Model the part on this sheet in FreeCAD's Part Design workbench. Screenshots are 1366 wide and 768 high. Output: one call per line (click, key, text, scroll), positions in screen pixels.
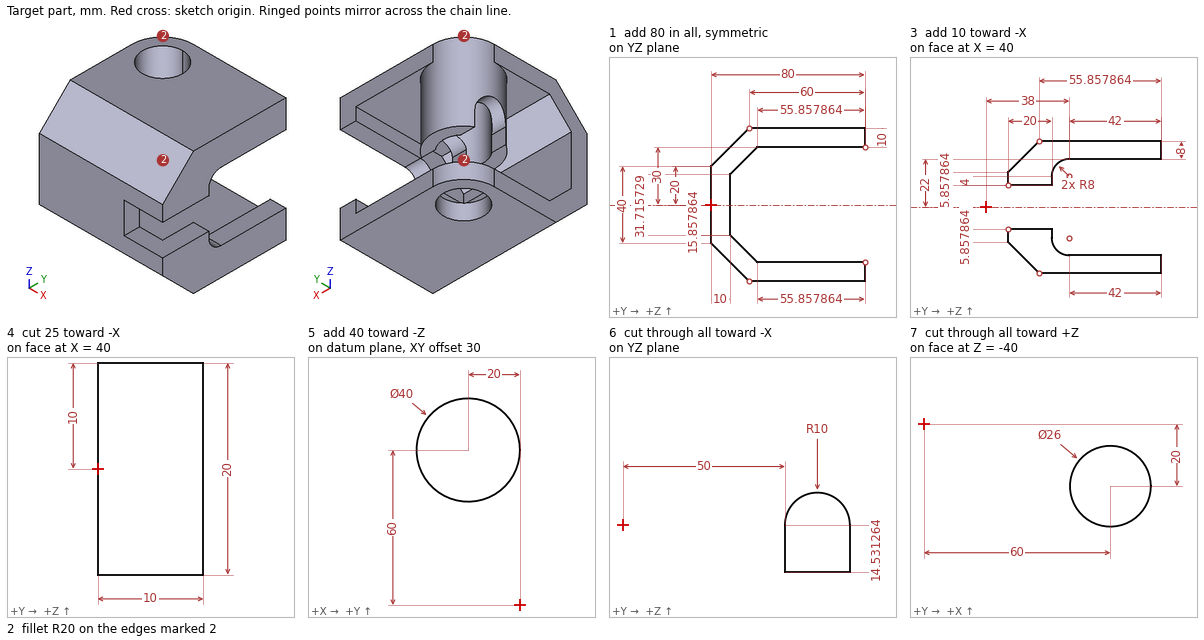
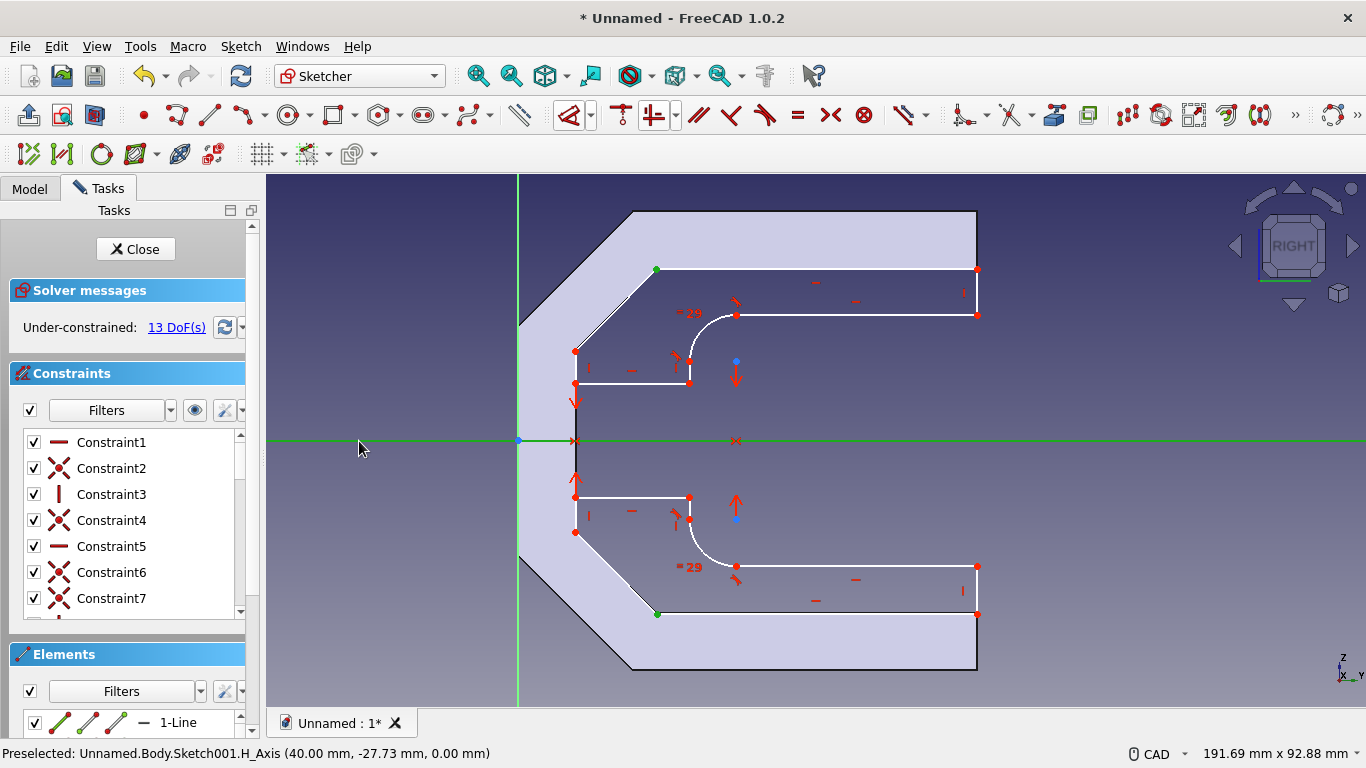
click(831, 116)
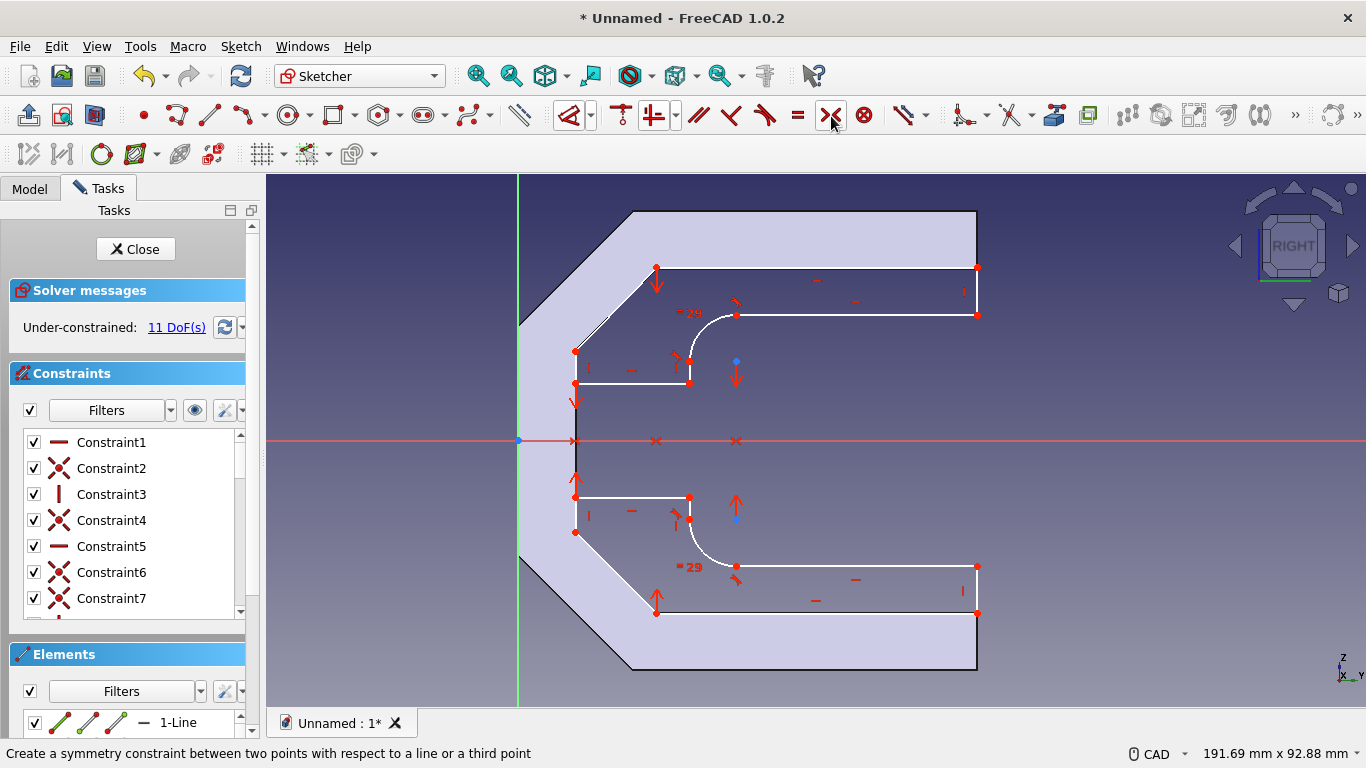
click(715, 320)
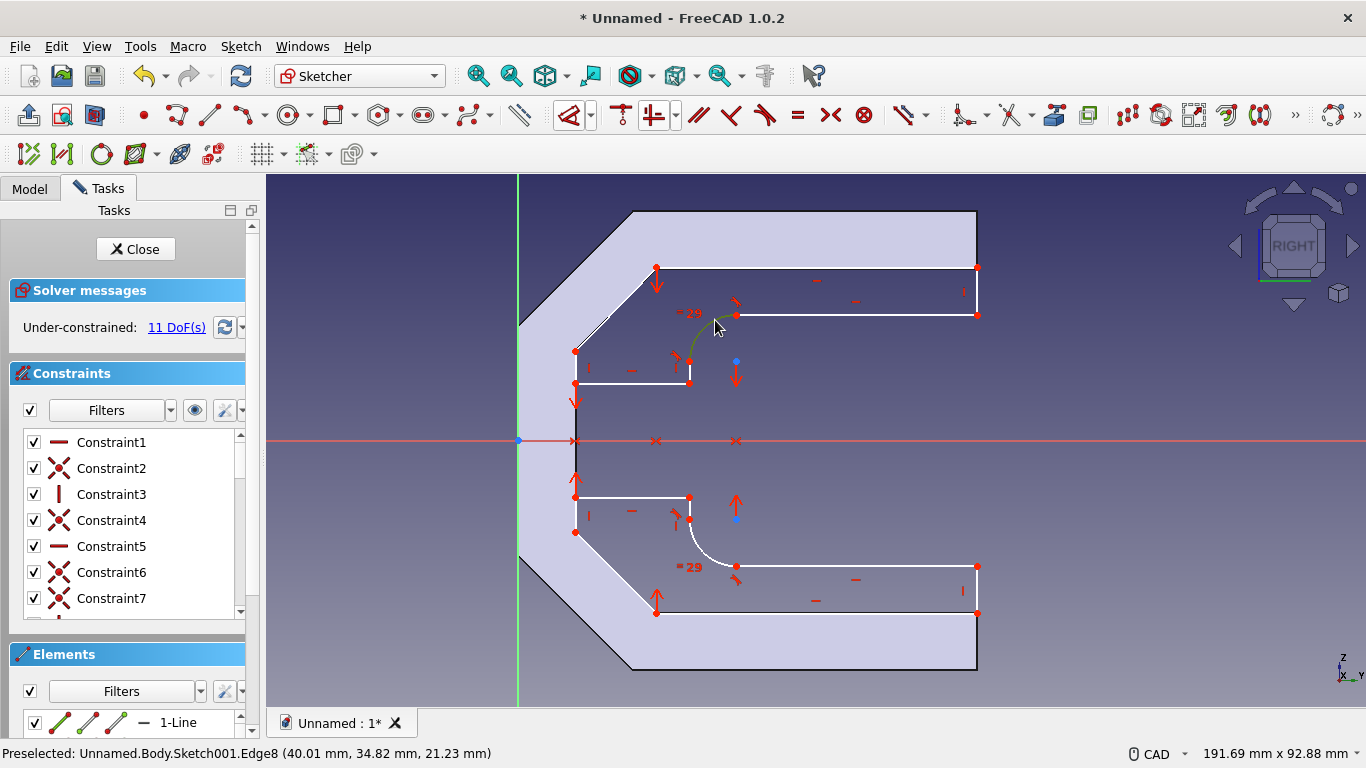
click(590, 116)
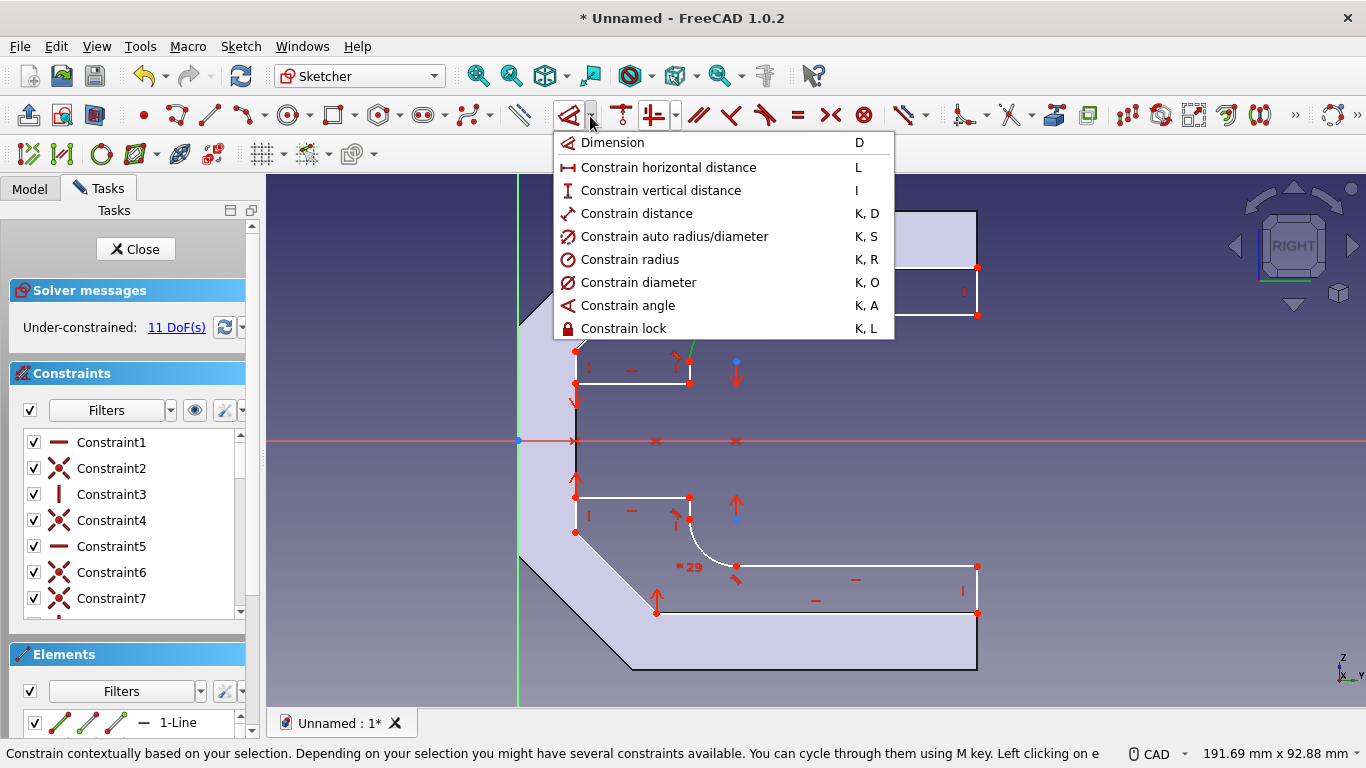
click(724, 260)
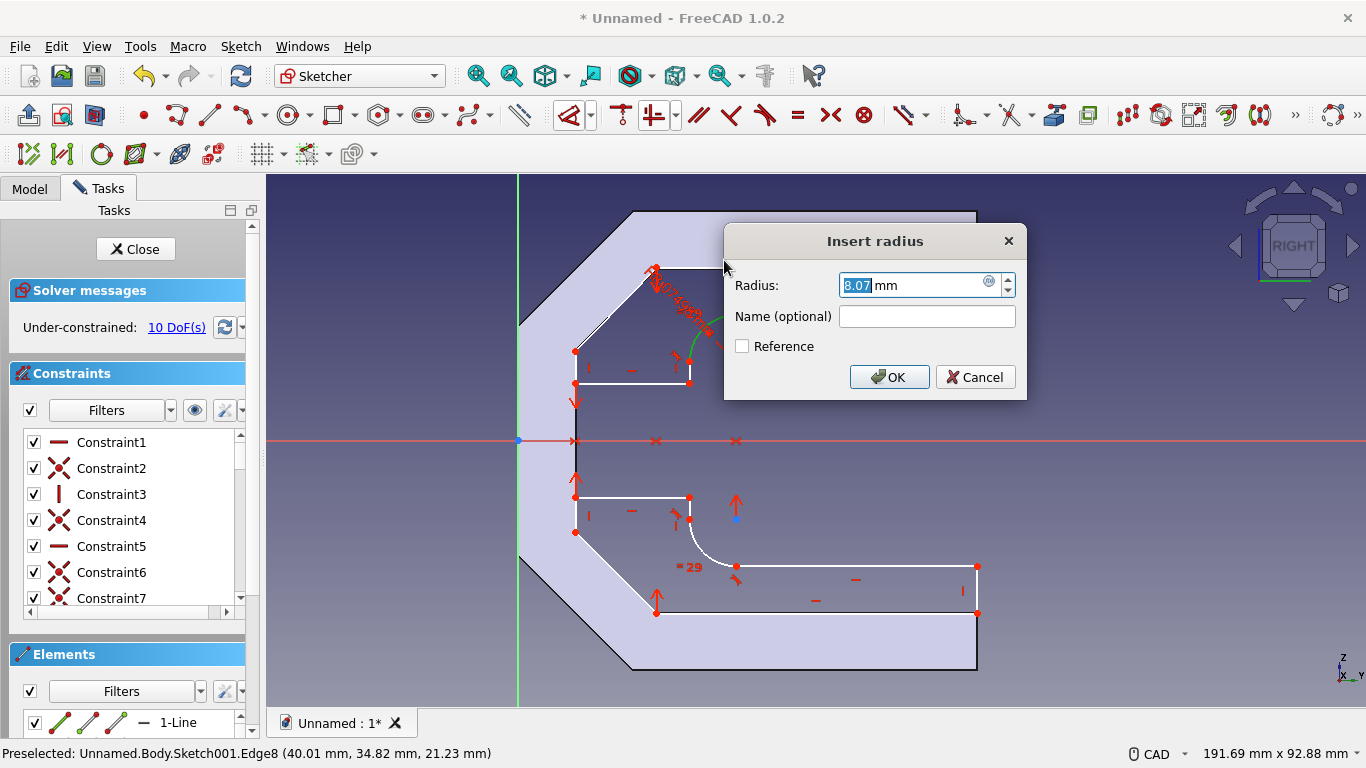
text(8)
key(Return)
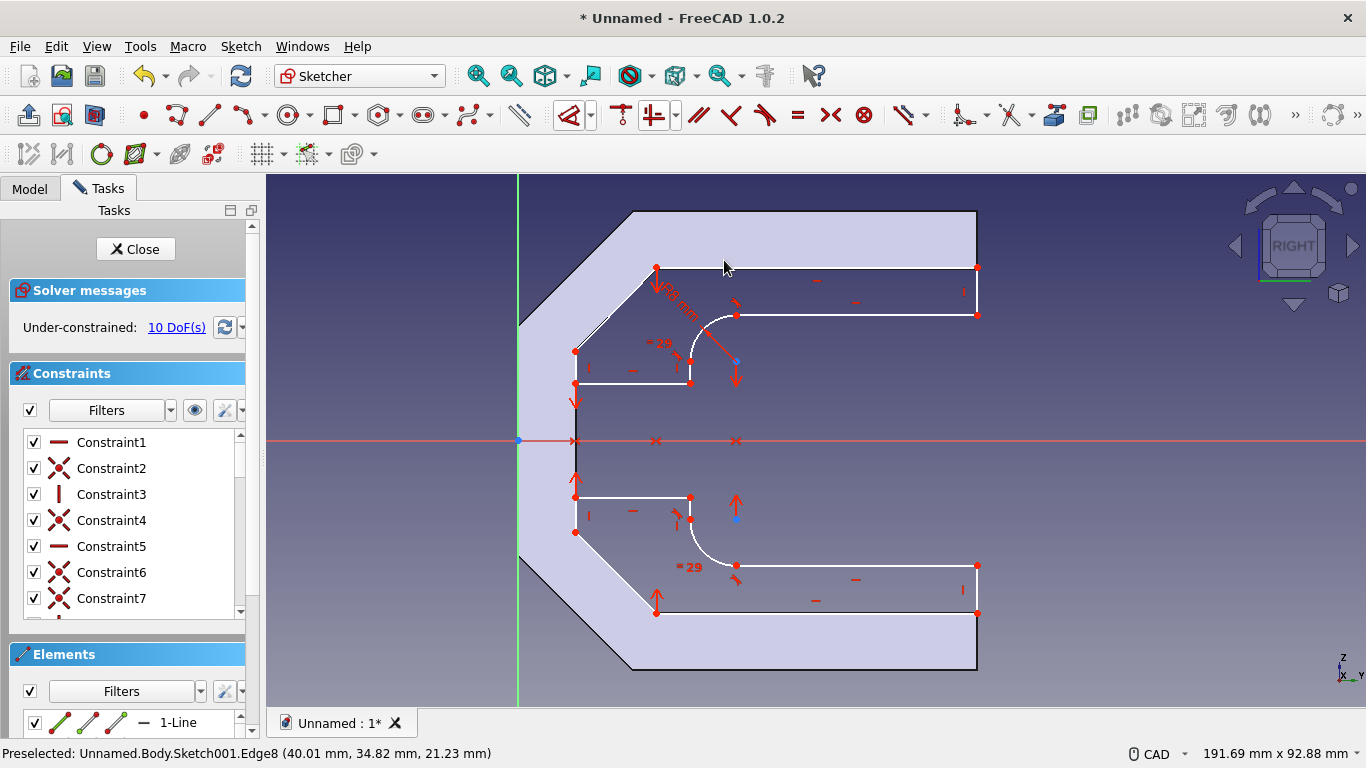
click(977, 301)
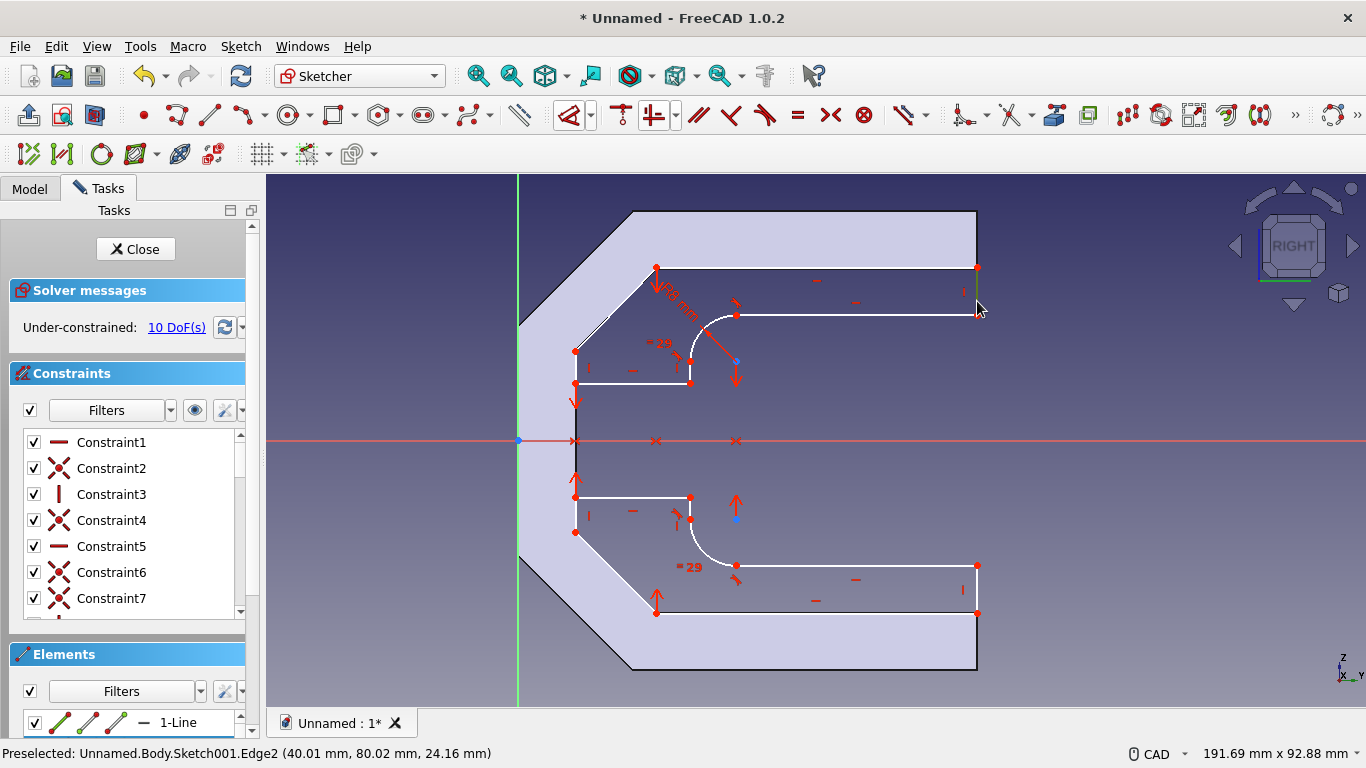
key(i)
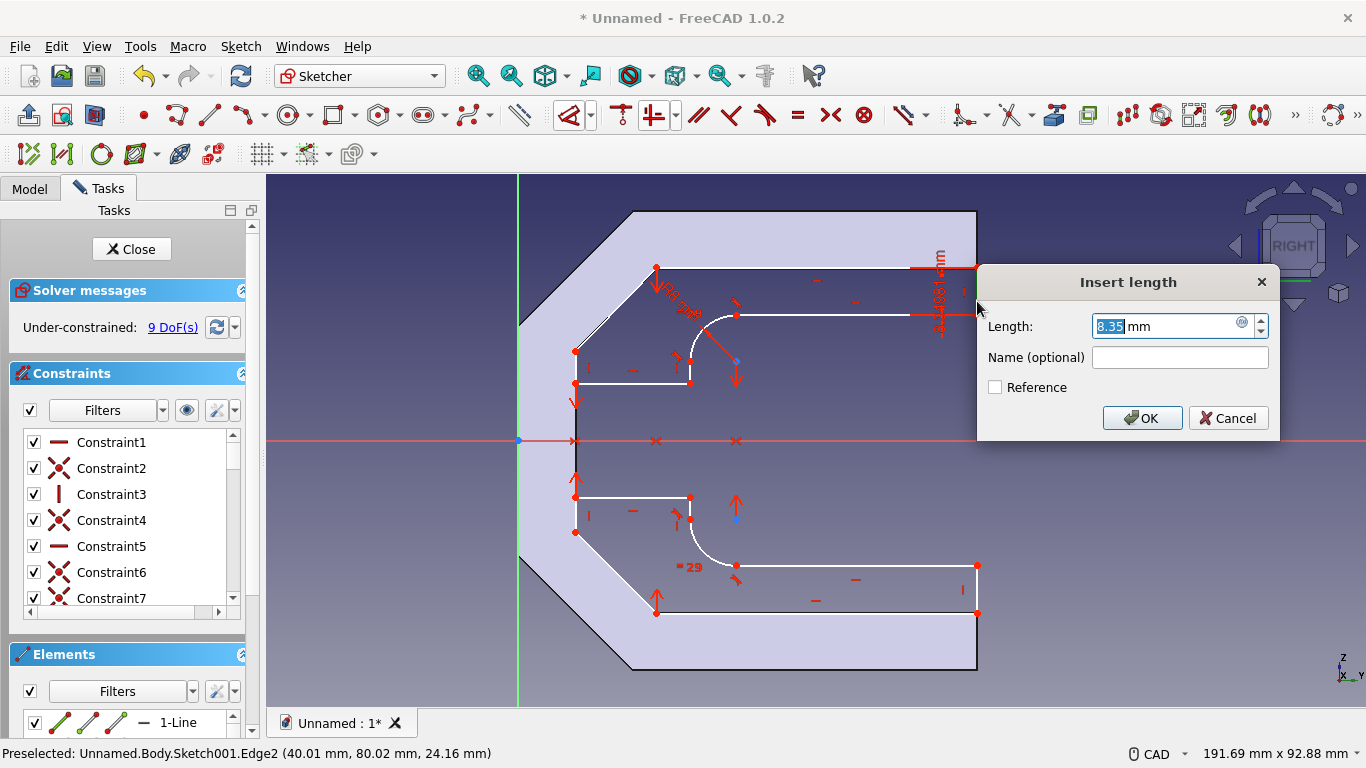
text(8)
key(Return)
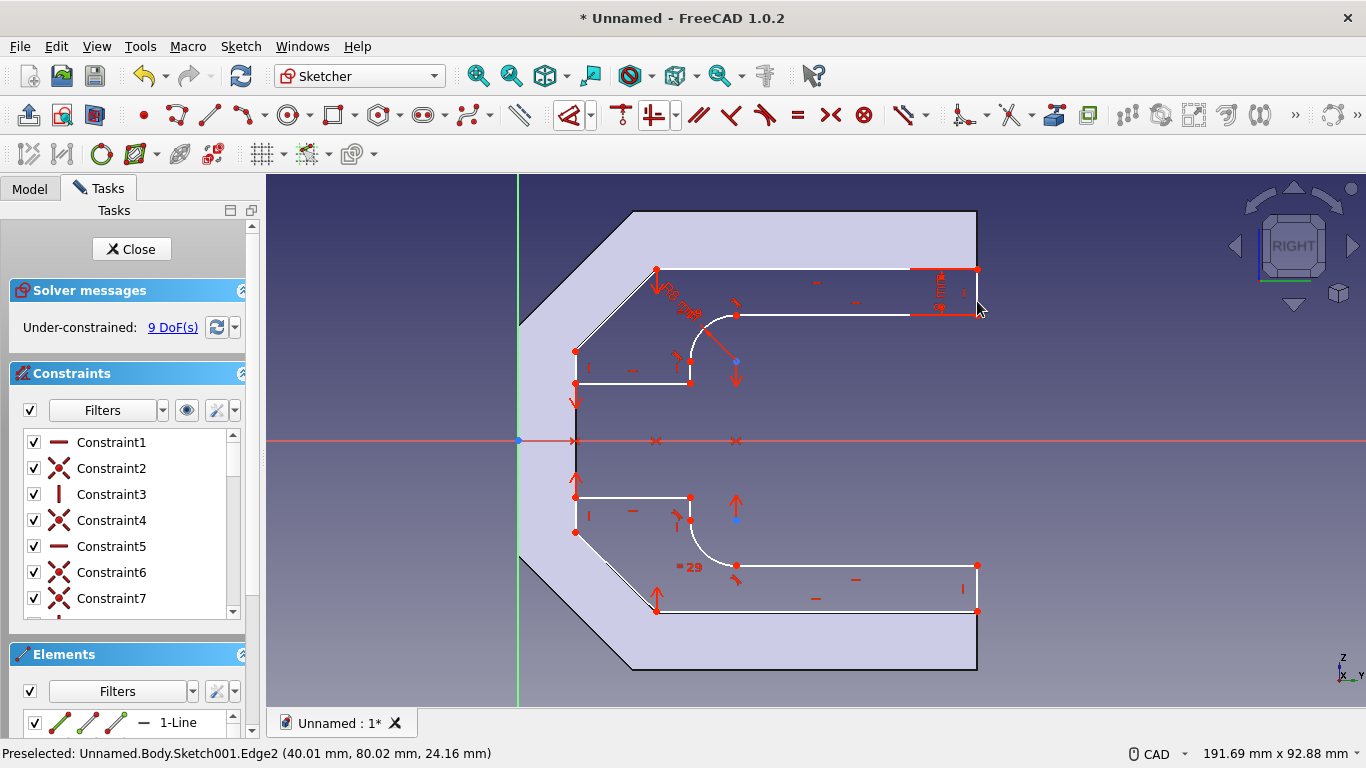
scroll(690, 373, up, 3)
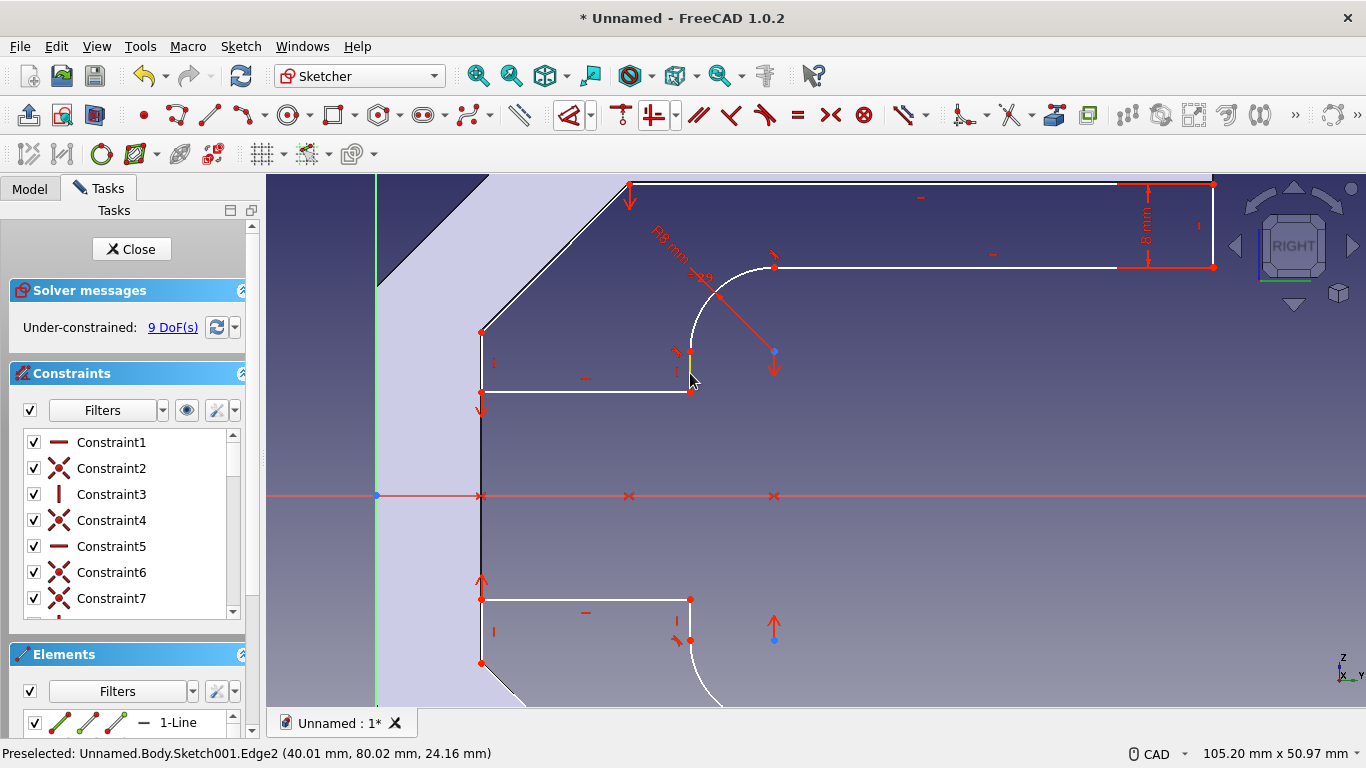
click(690, 372)